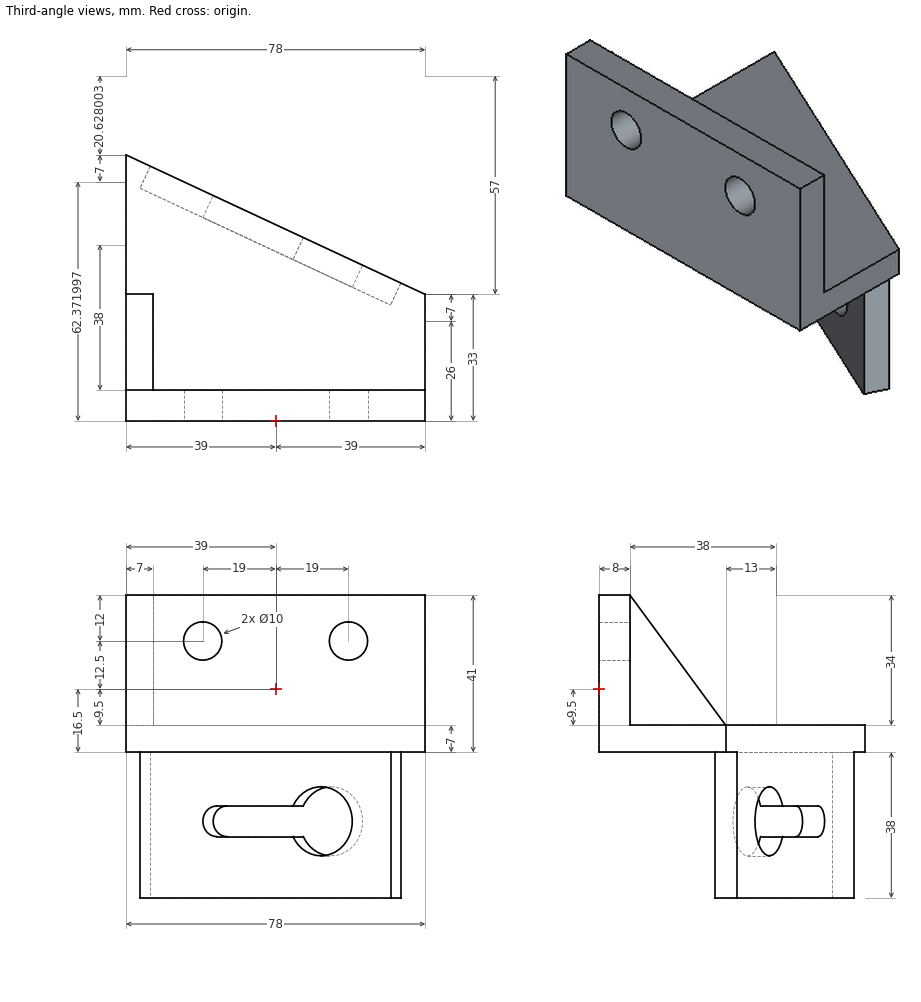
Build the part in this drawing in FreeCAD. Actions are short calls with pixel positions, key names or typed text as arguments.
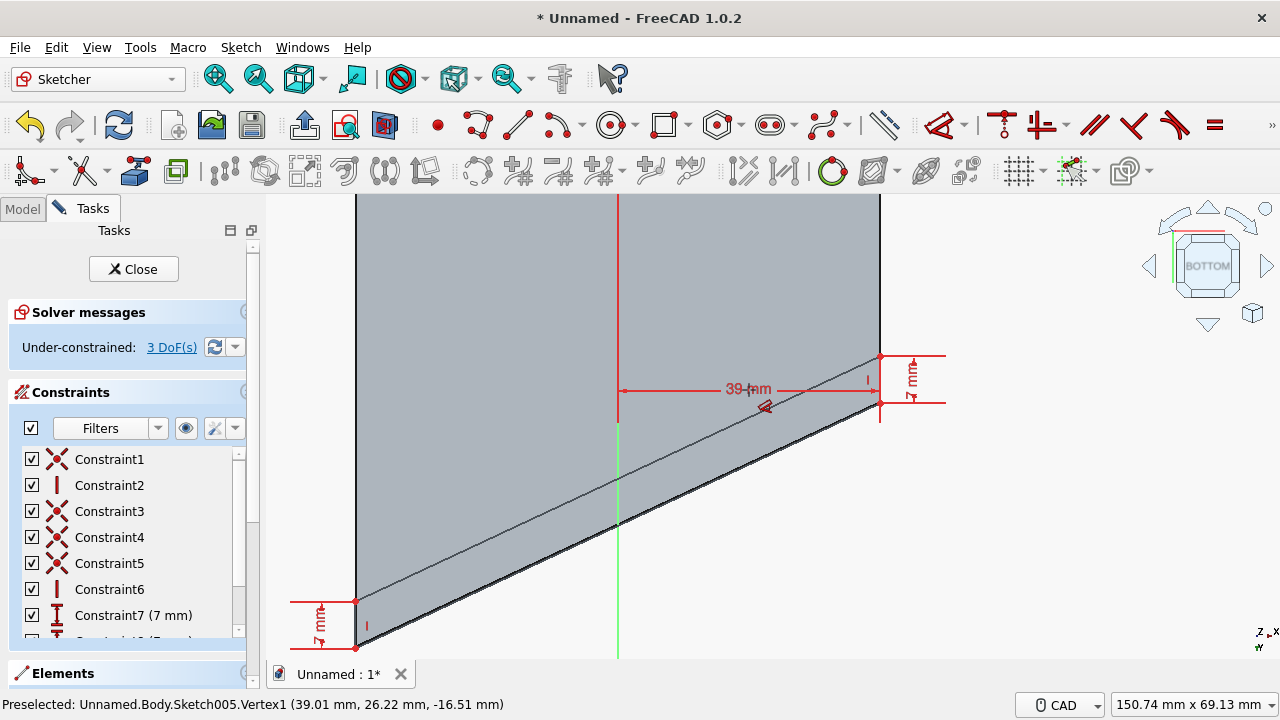
click(880, 356)
click(914, 289)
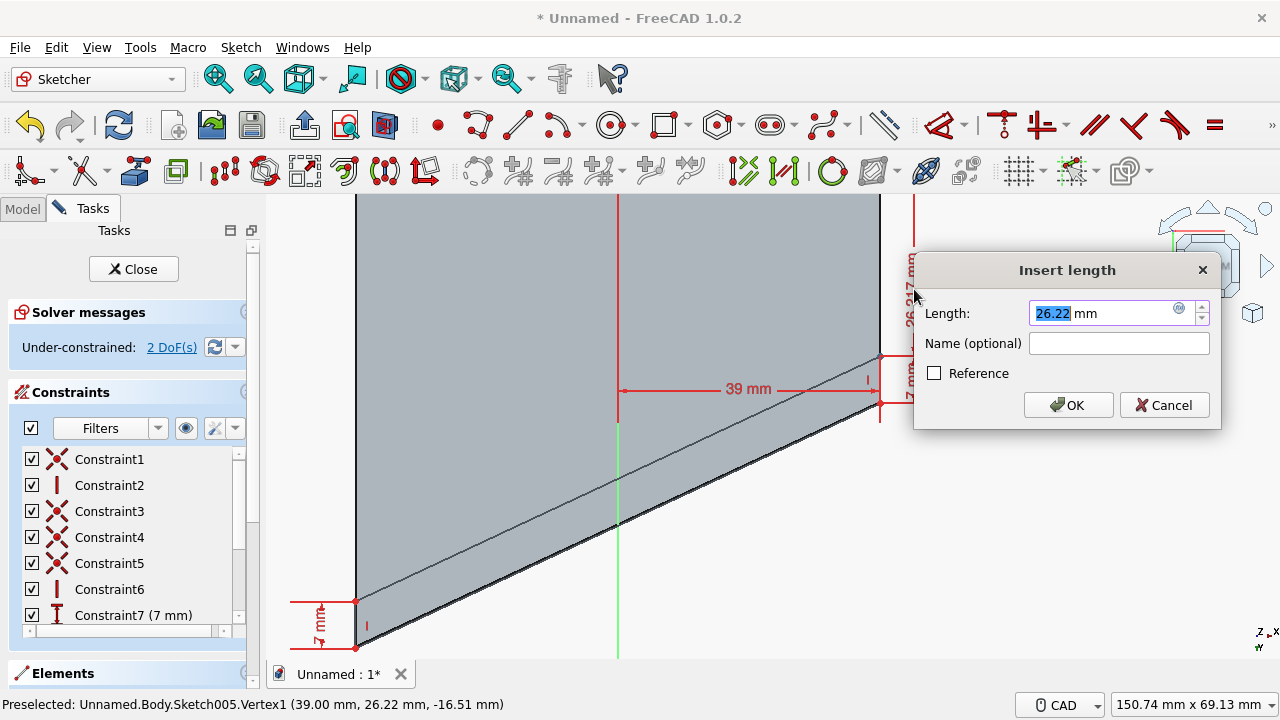
text(26)
key(Return)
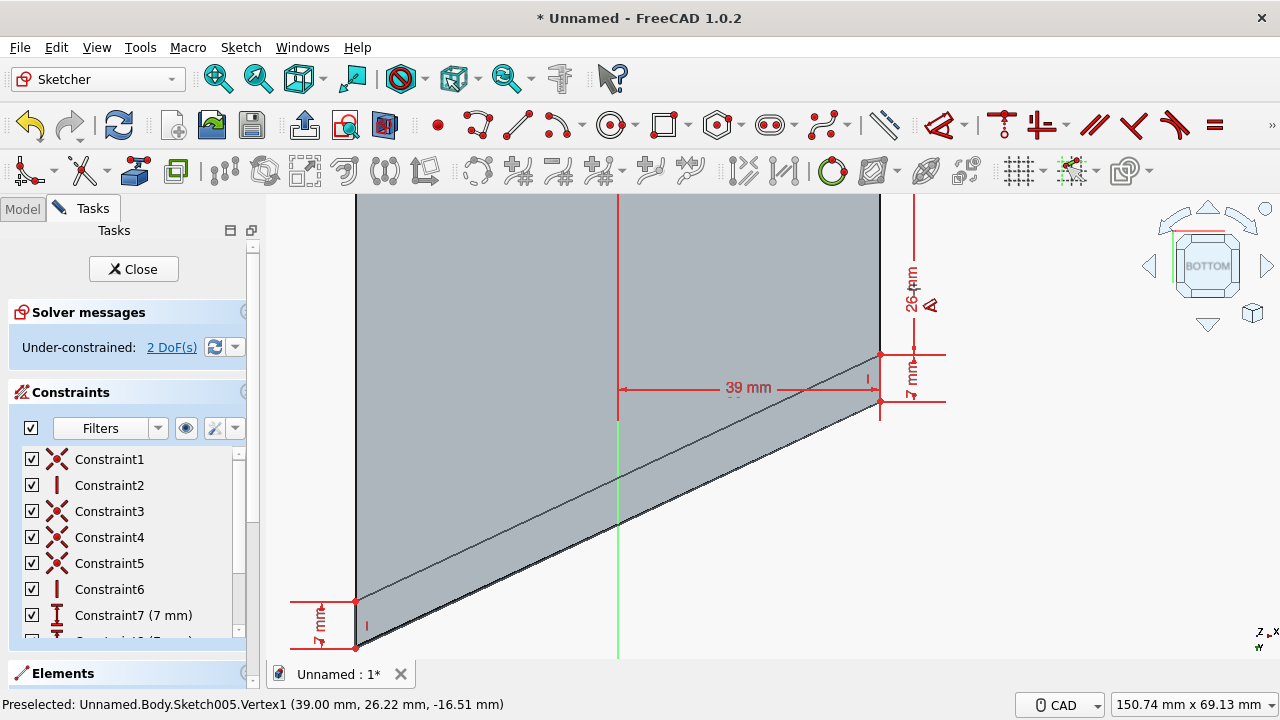
click(355, 602)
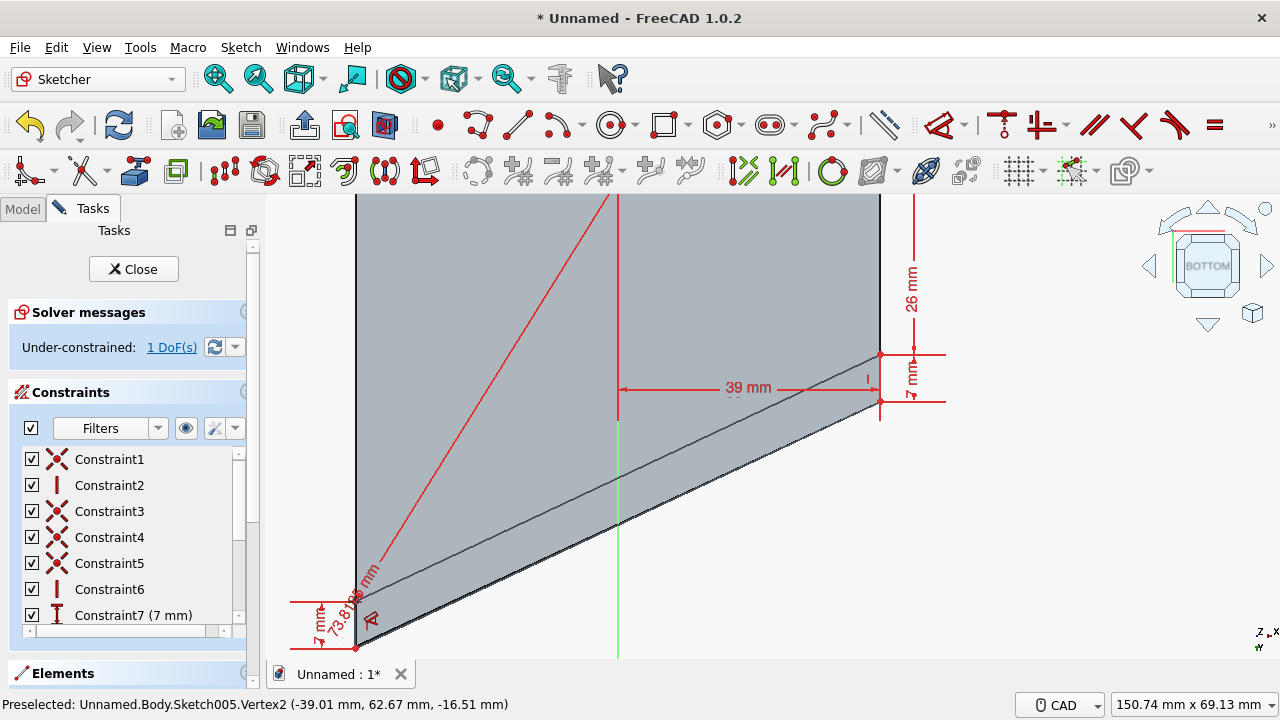
key(Escape)
key(Escape)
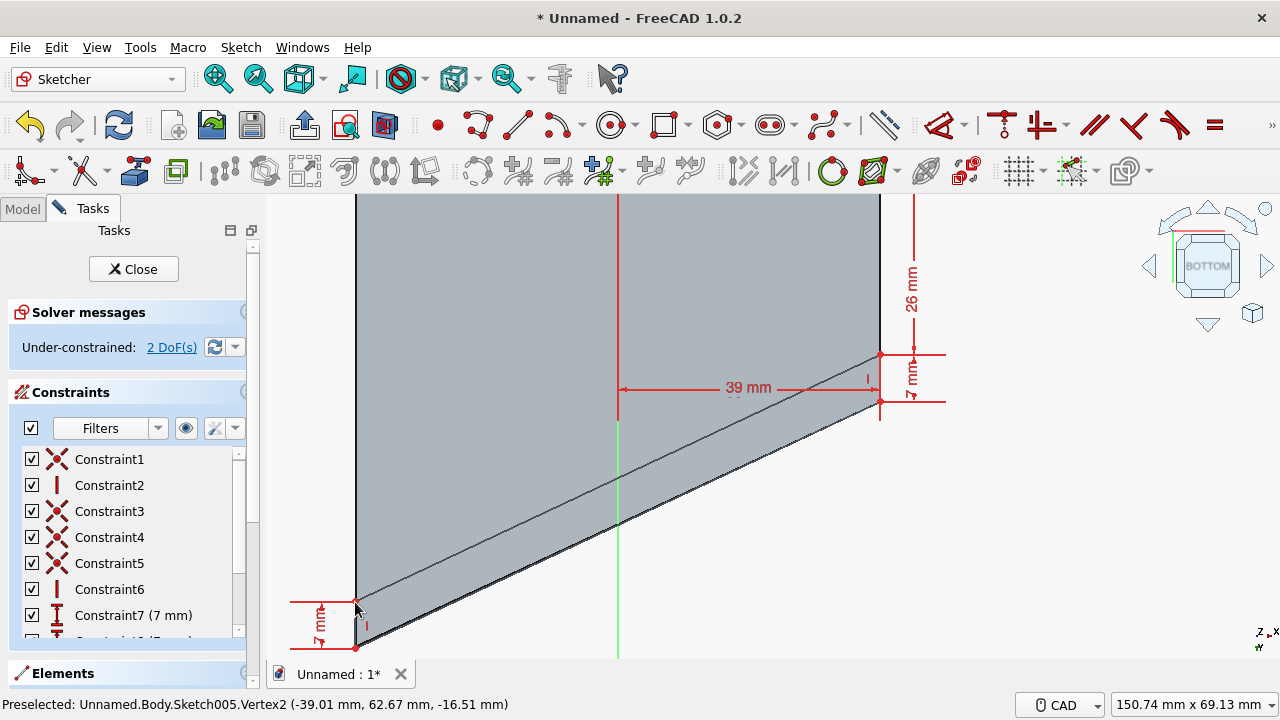
click(355, 602)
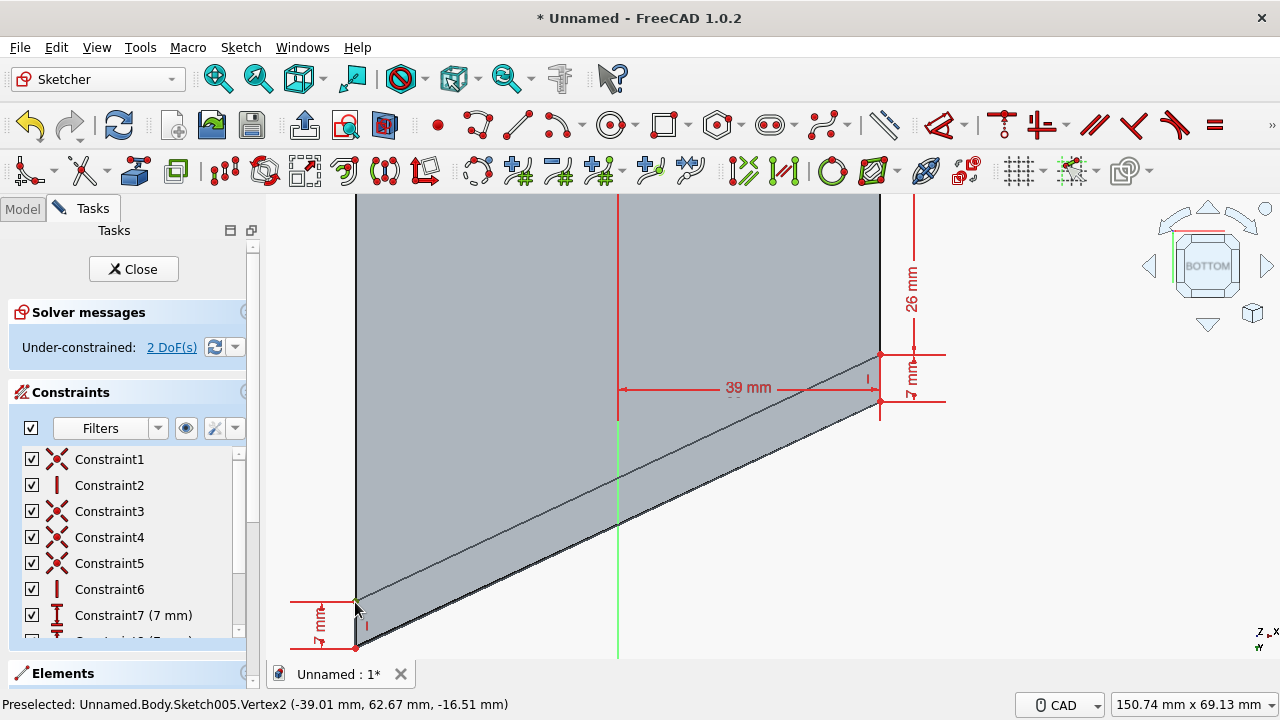
key(l)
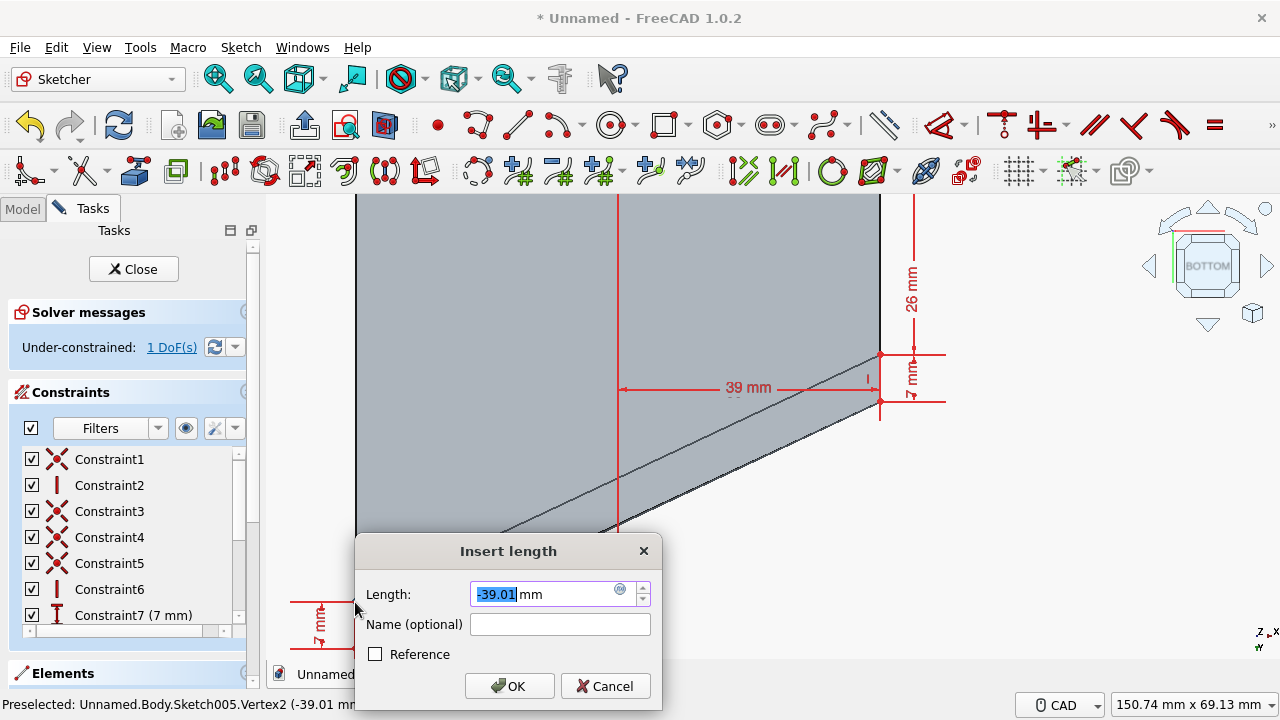
text(-39)
key(Return)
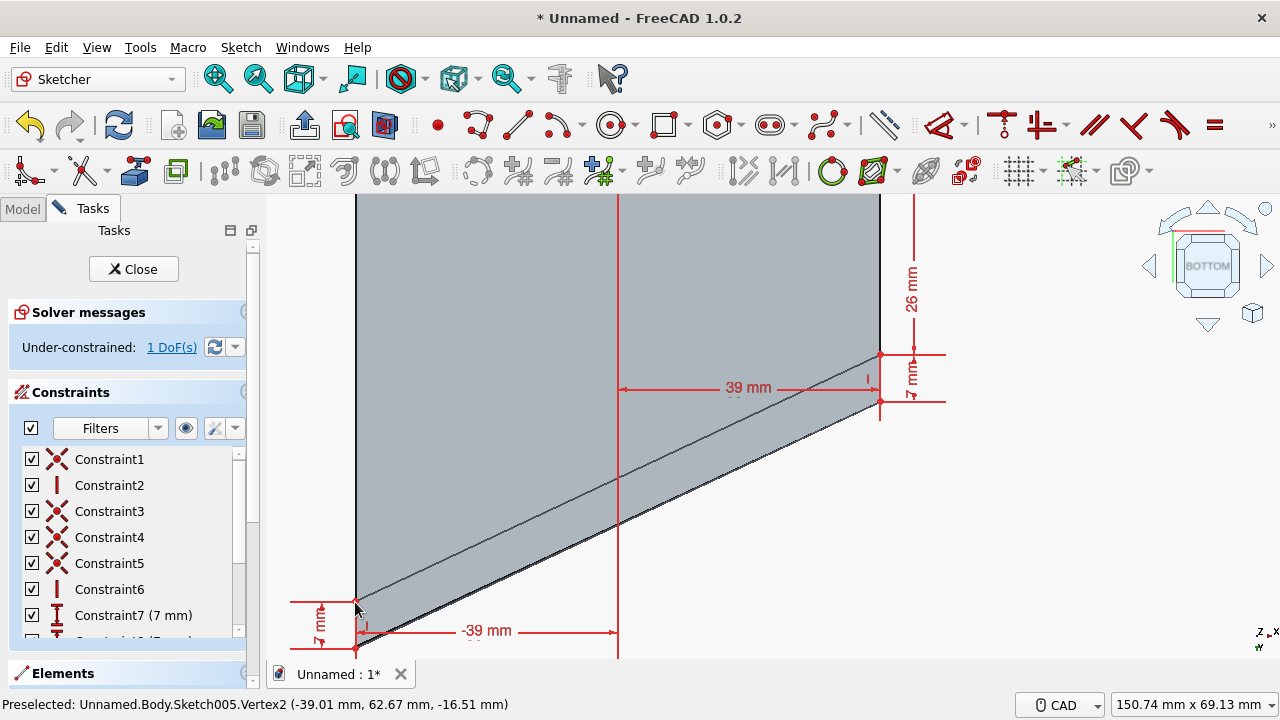
click(356, 602)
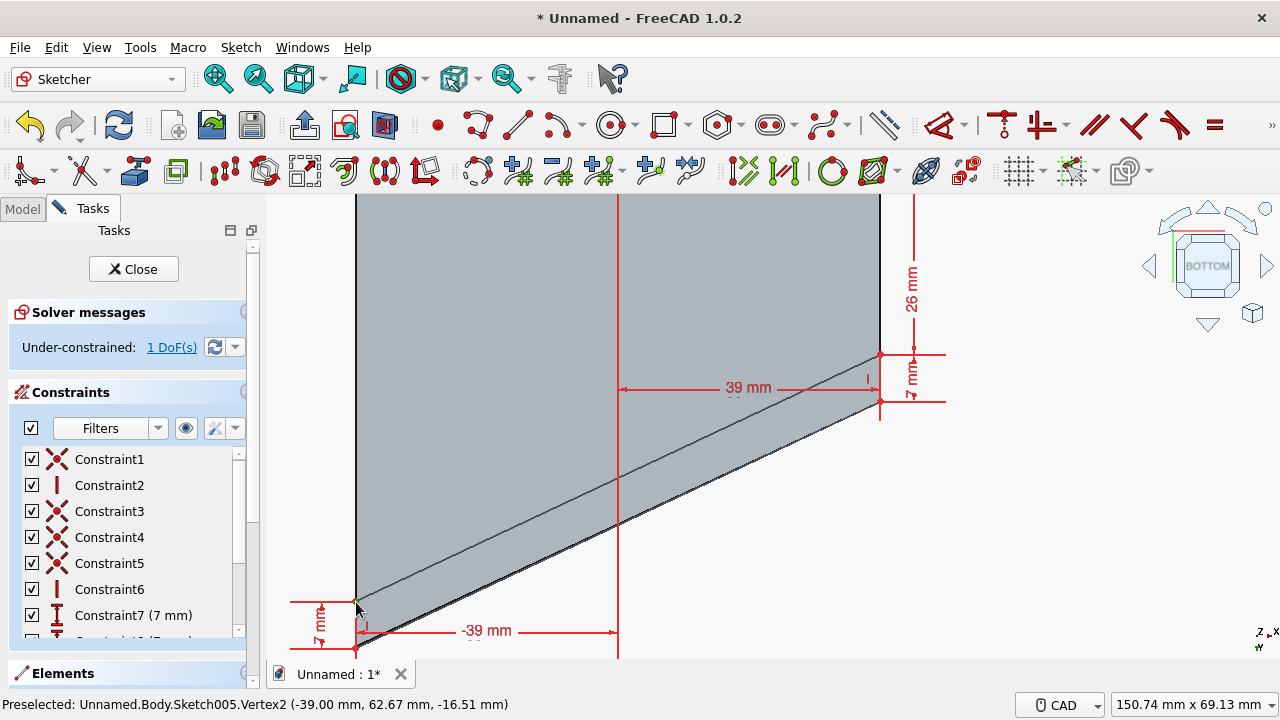
click(966, 126)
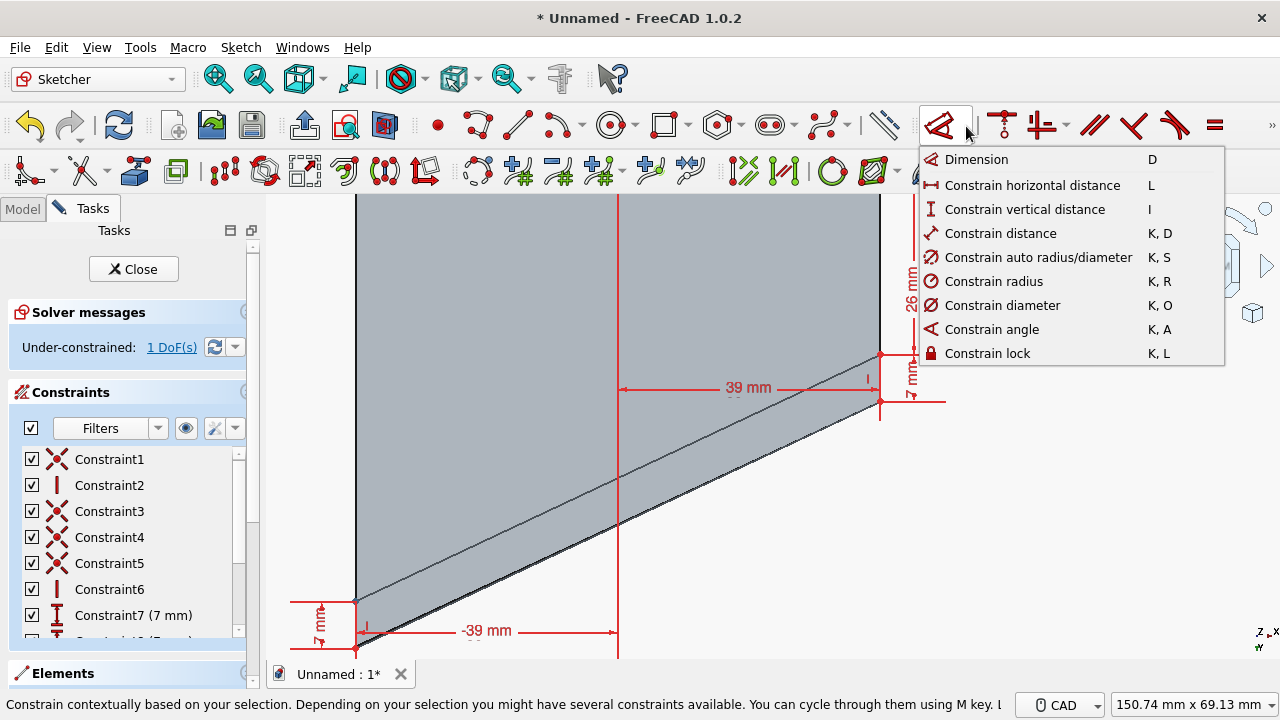
click(1072, 209)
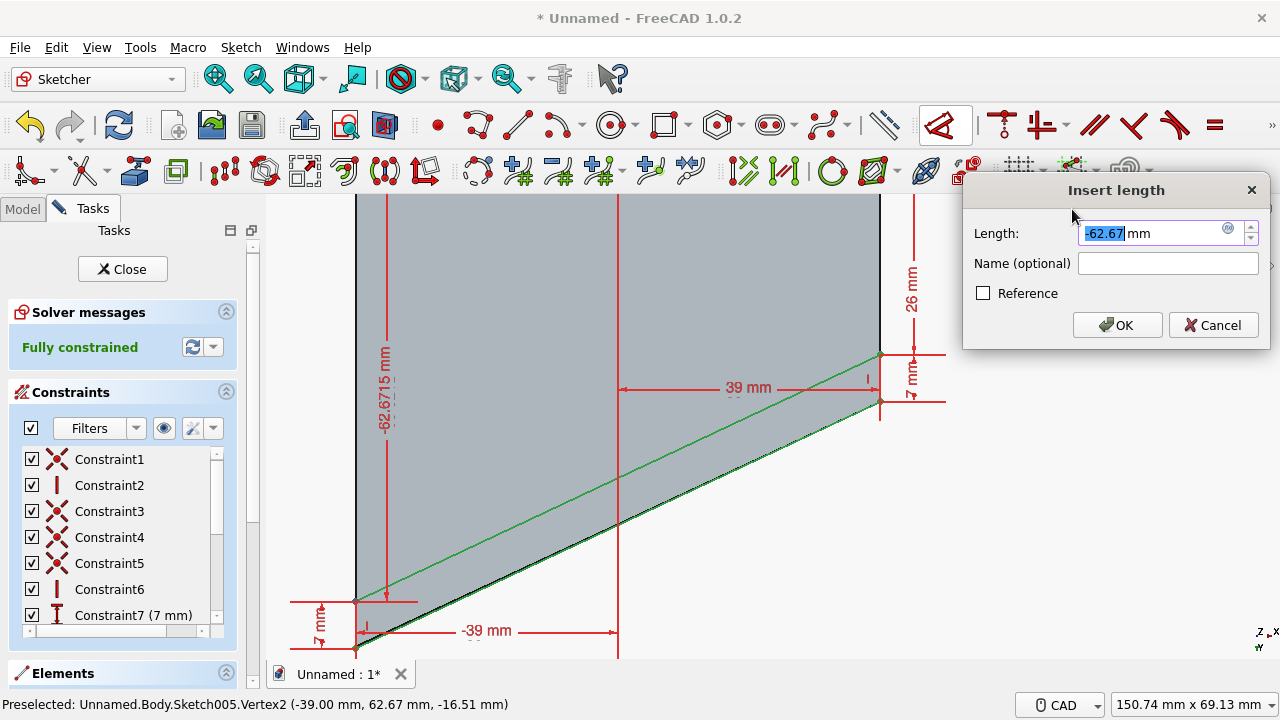
text(-62.371997)
key(Return)